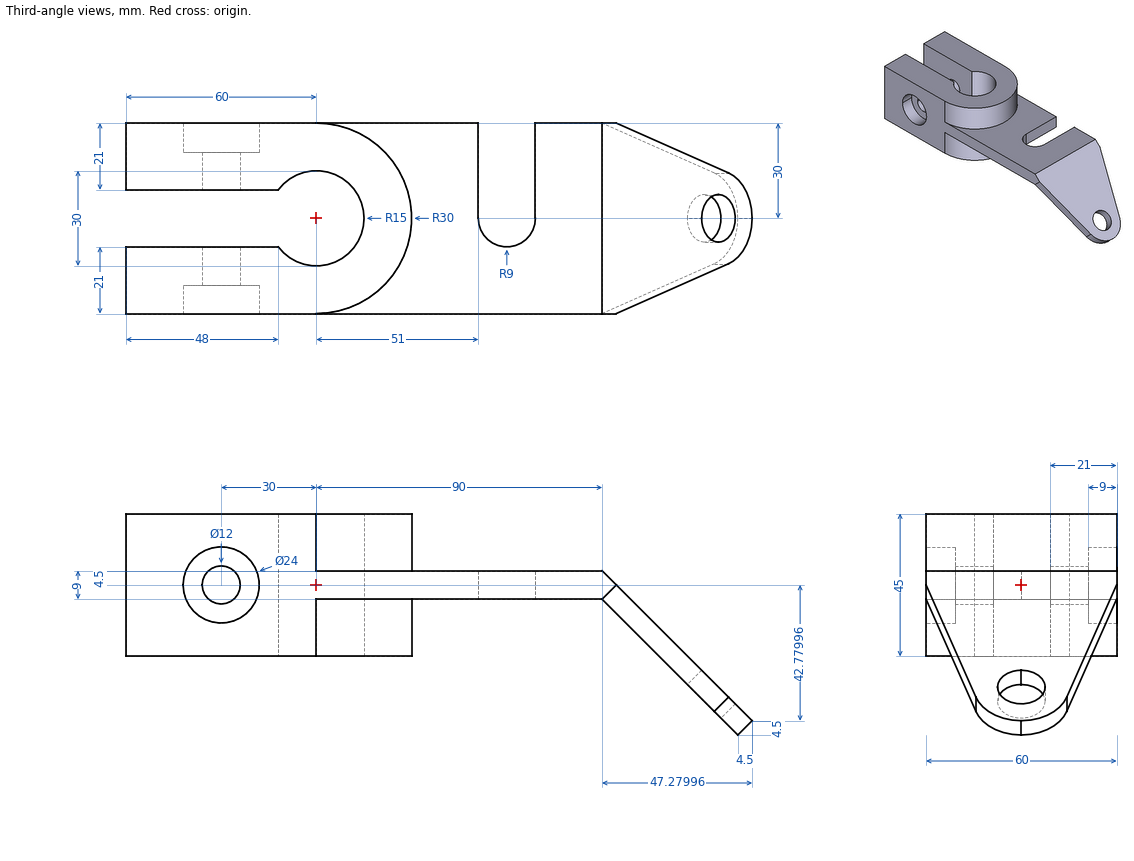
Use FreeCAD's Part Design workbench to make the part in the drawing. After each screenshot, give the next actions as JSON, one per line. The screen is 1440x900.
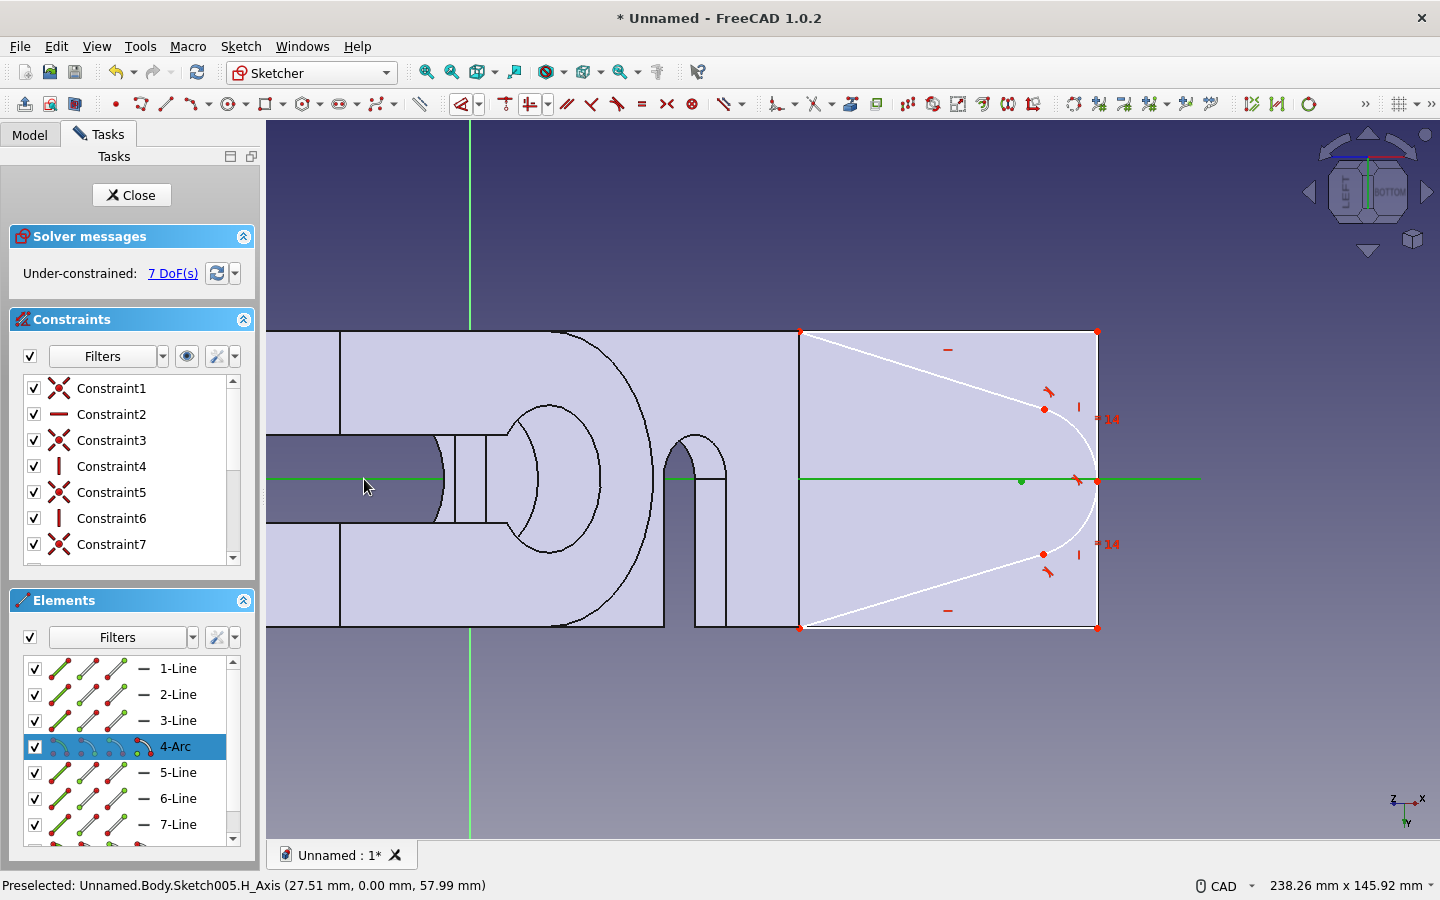
{"action": "left_click", "coordinate": [505, 104]}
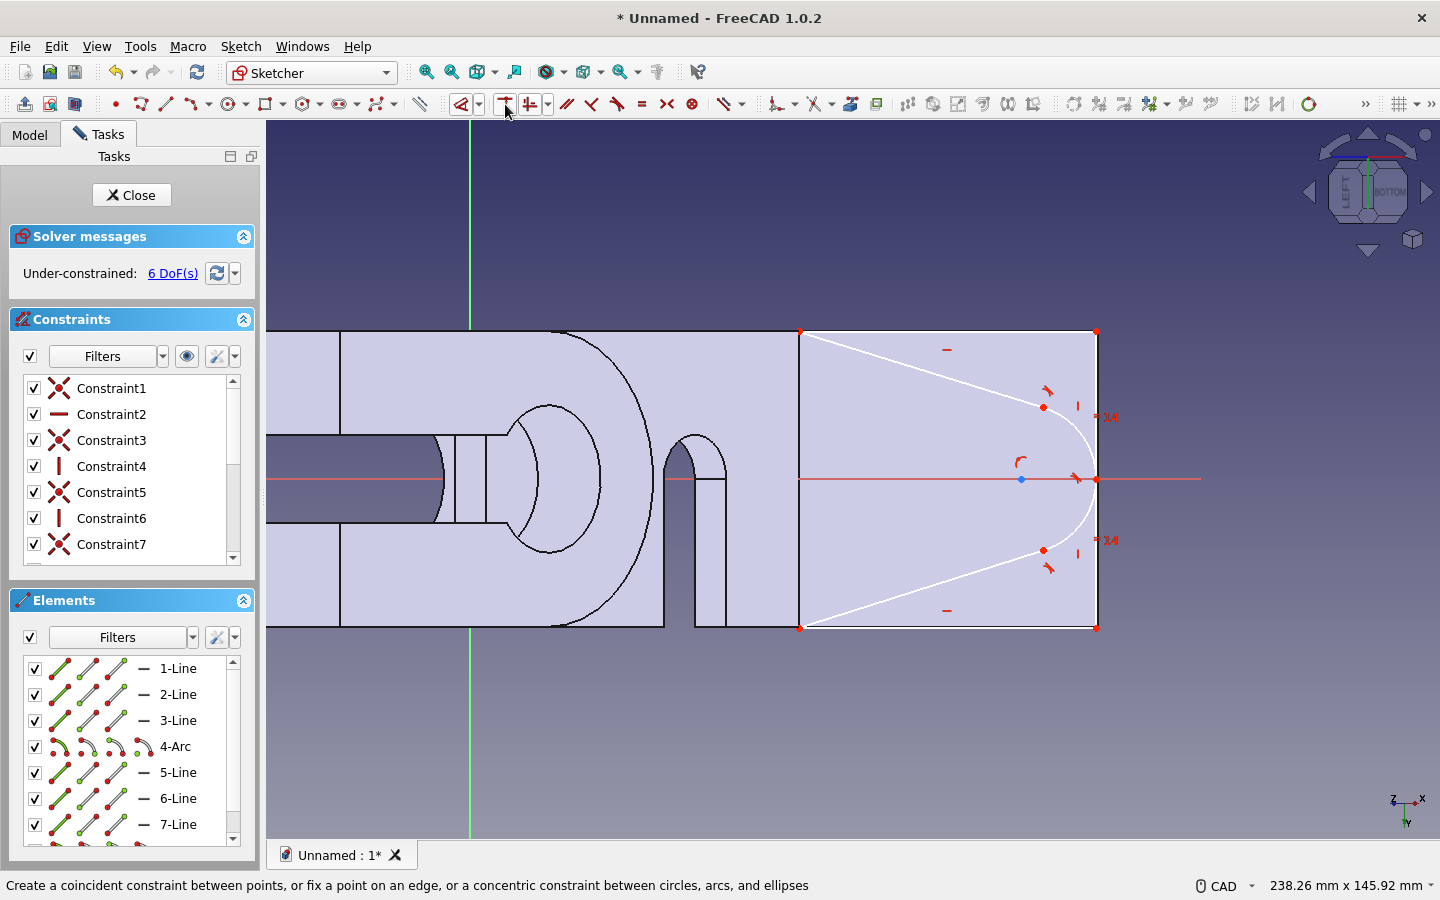
{"action": "left_click", "coordinate": [1069, 537]}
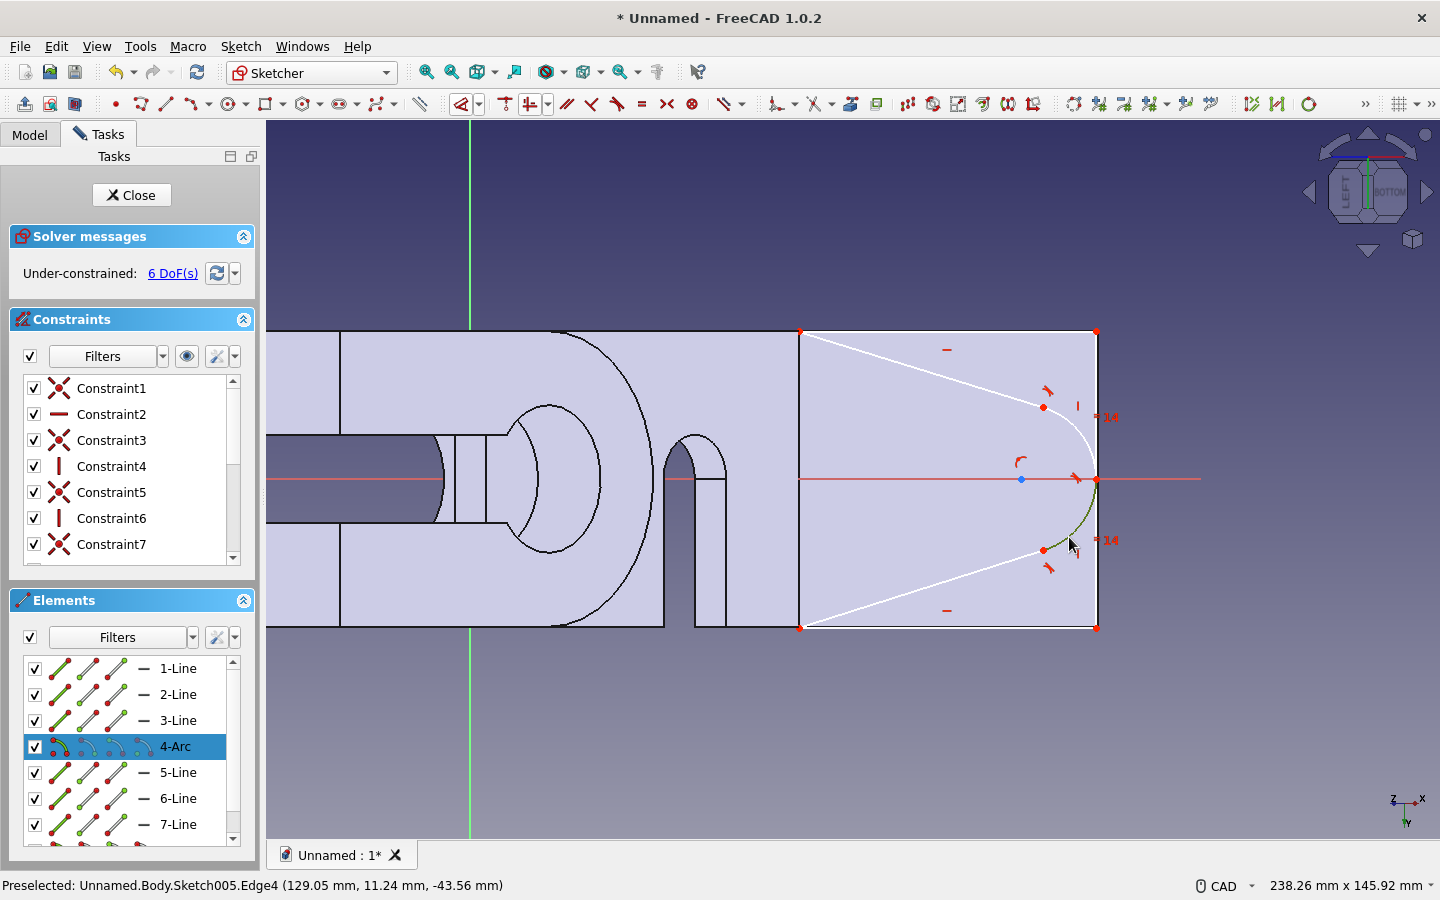
{"action": "left_click", "coordinate": [478, 104]}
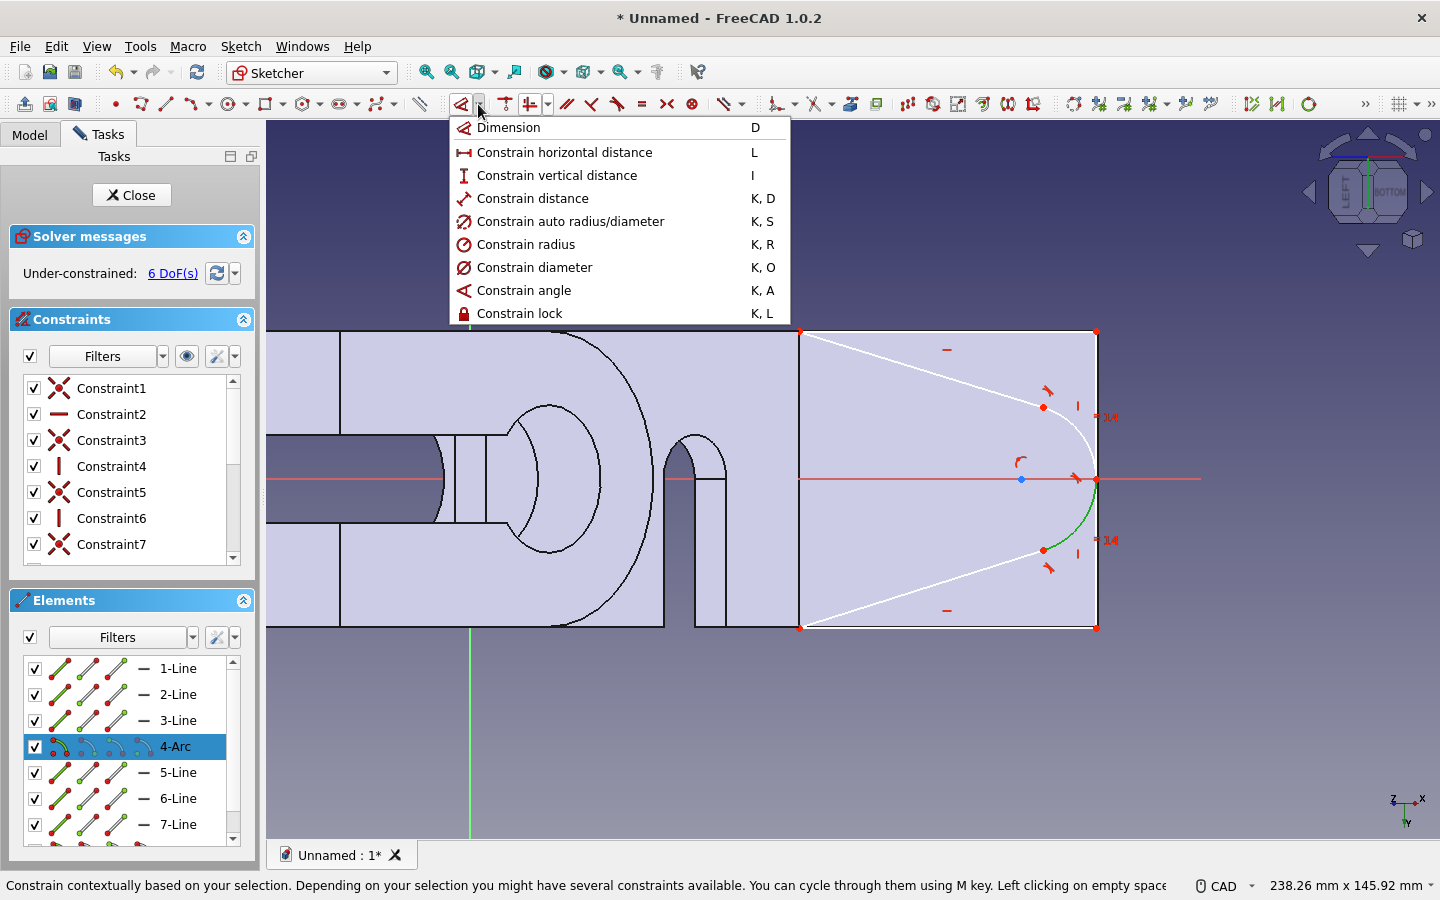
{"action": "left_click", "coordinate": [620, 244]}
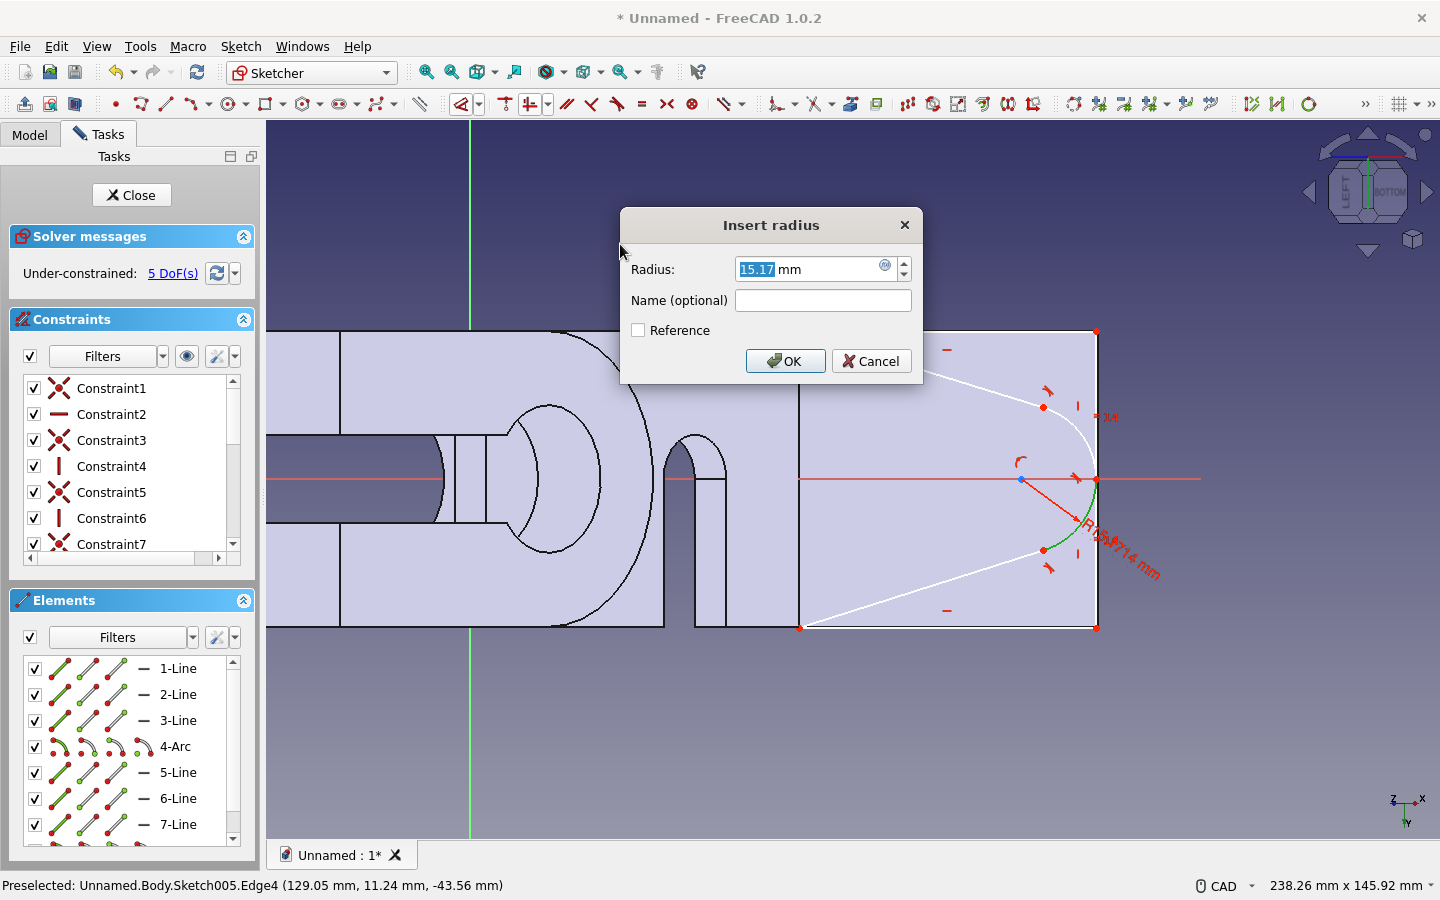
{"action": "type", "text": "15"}
{"action": "key", "text": "Return"}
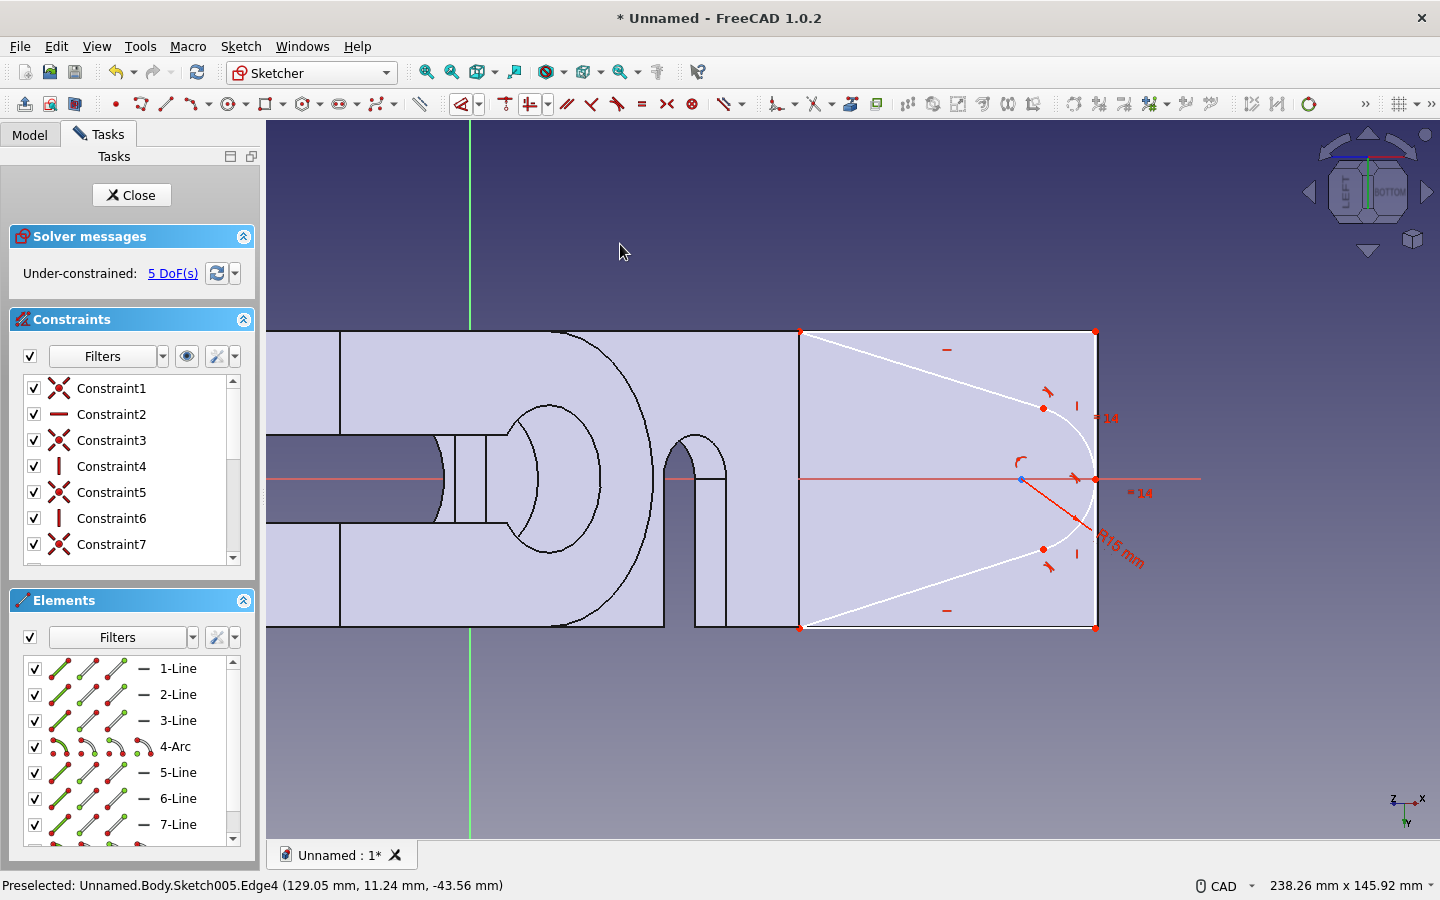
{"action": "left_click", "coordinate": [1095, 583]}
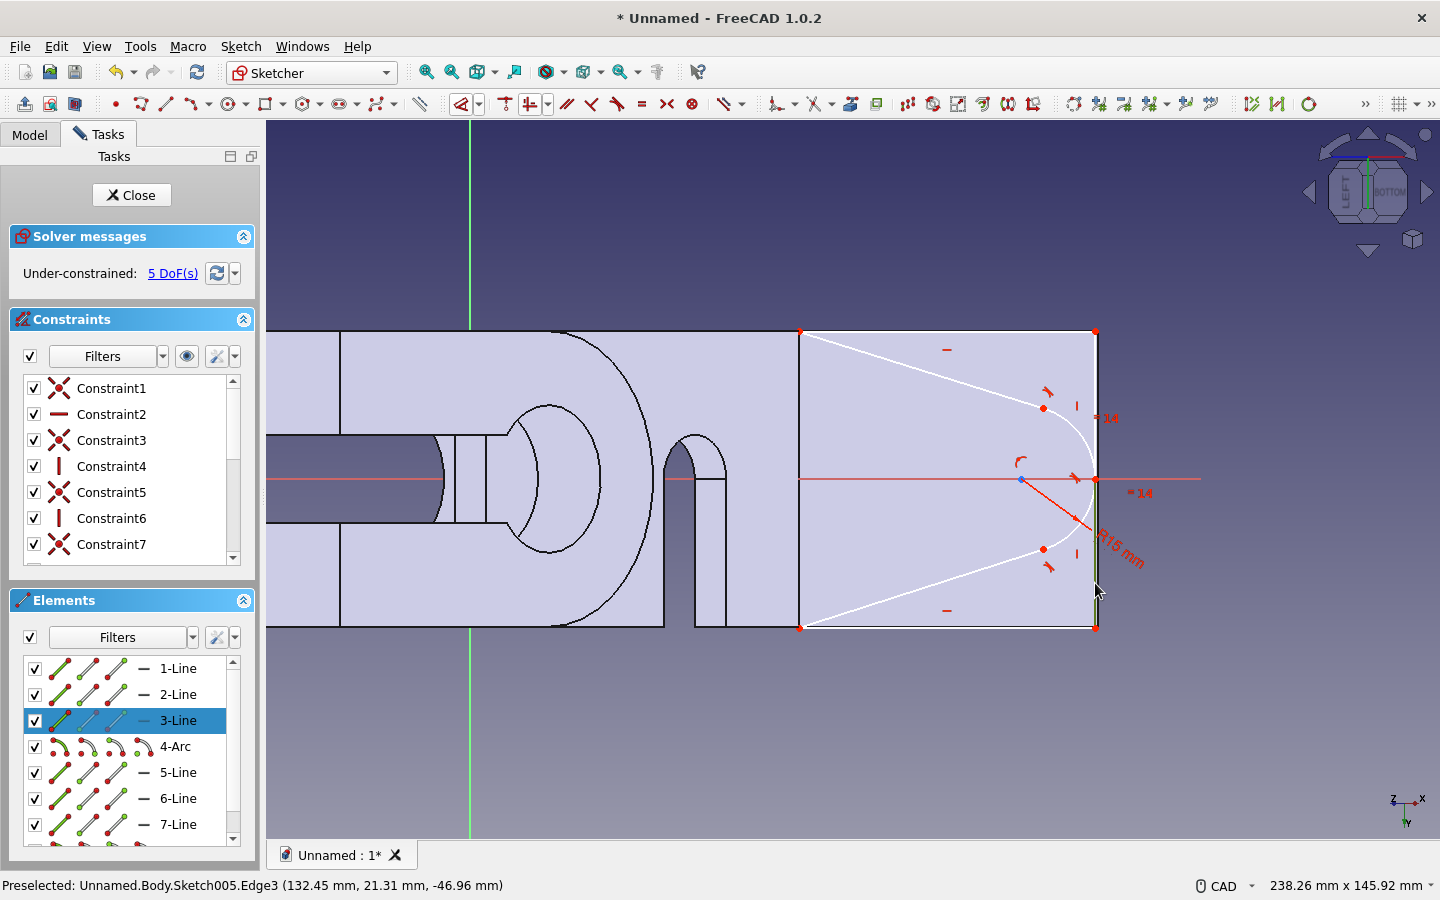
{"action": "left_click", "coordinate": [478, 104]}